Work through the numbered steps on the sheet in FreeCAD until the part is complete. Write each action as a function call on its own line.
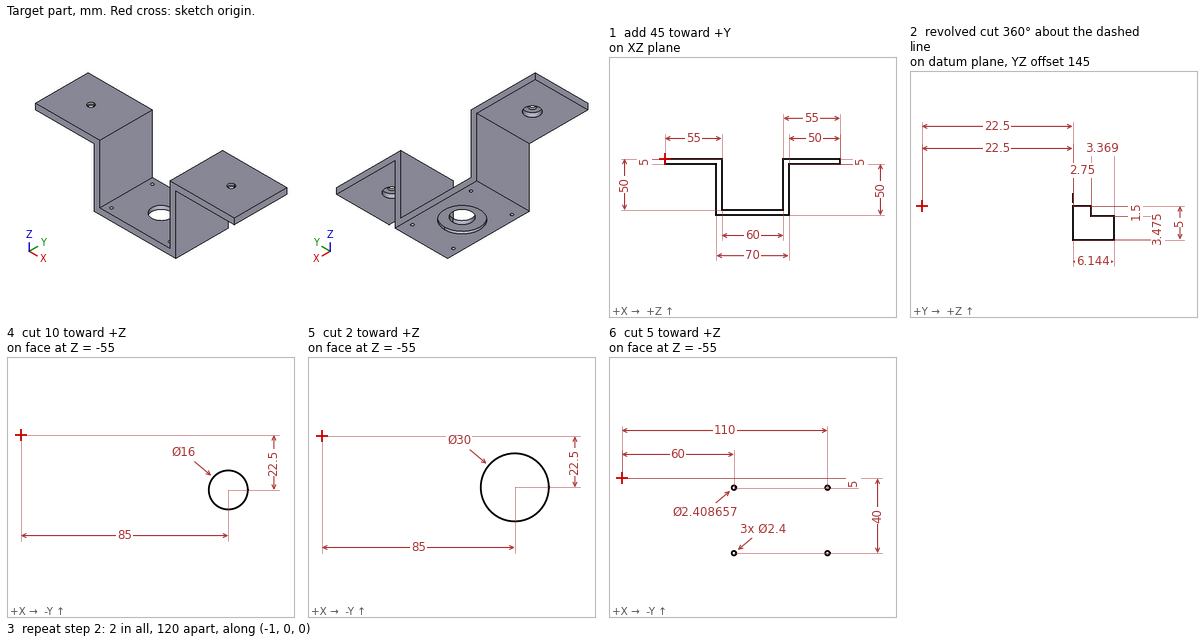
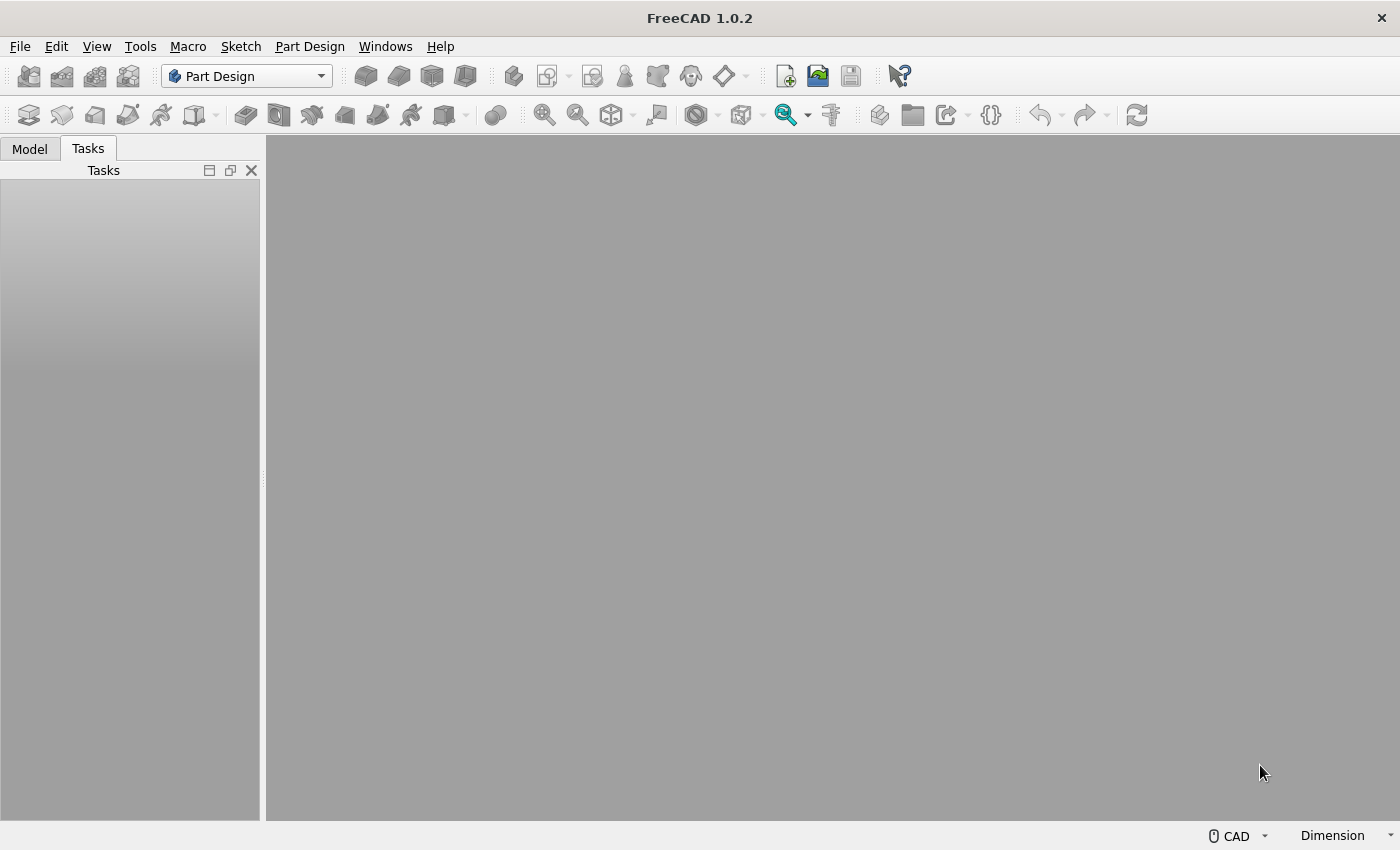
click(785, 76)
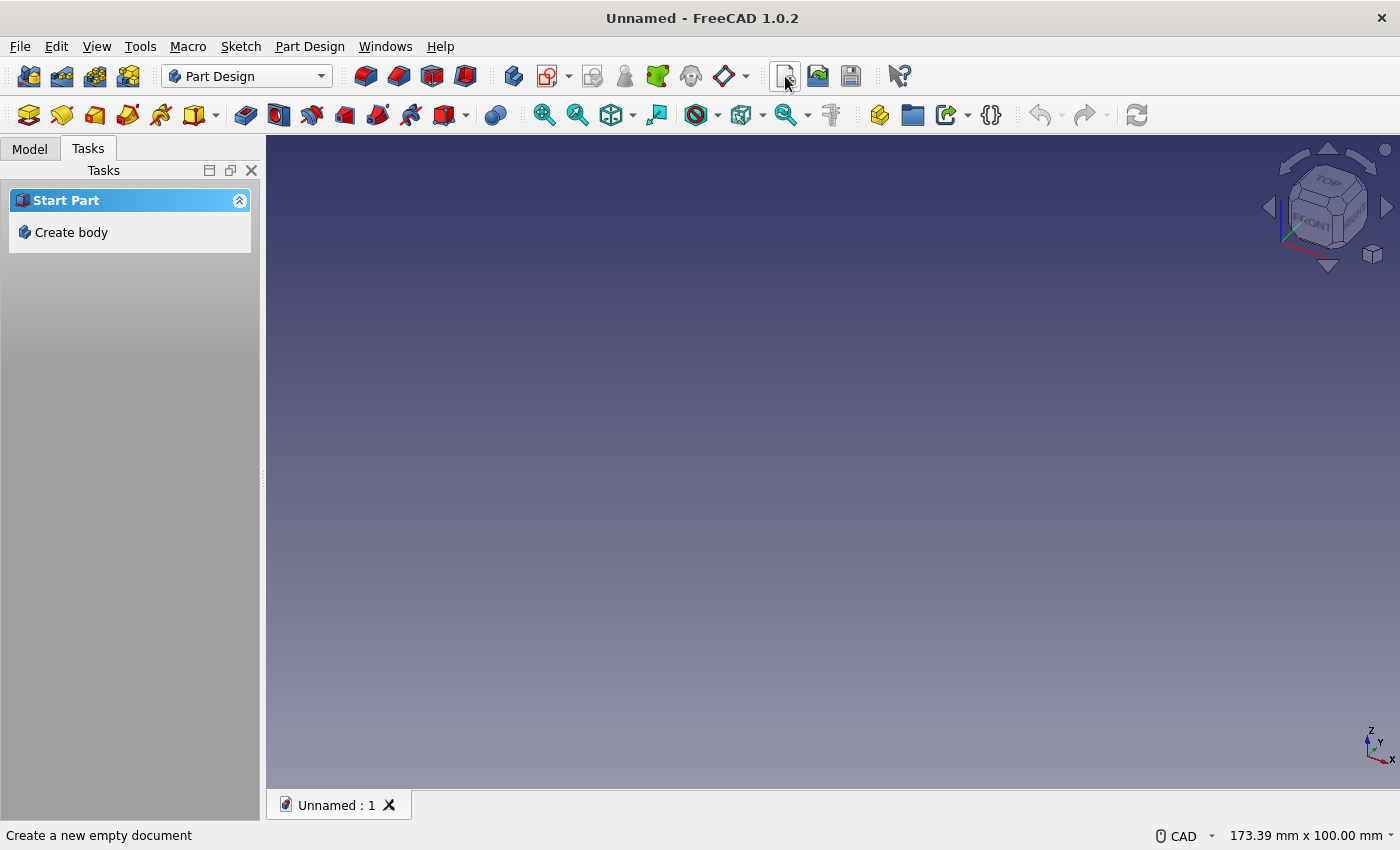
click(546, 76)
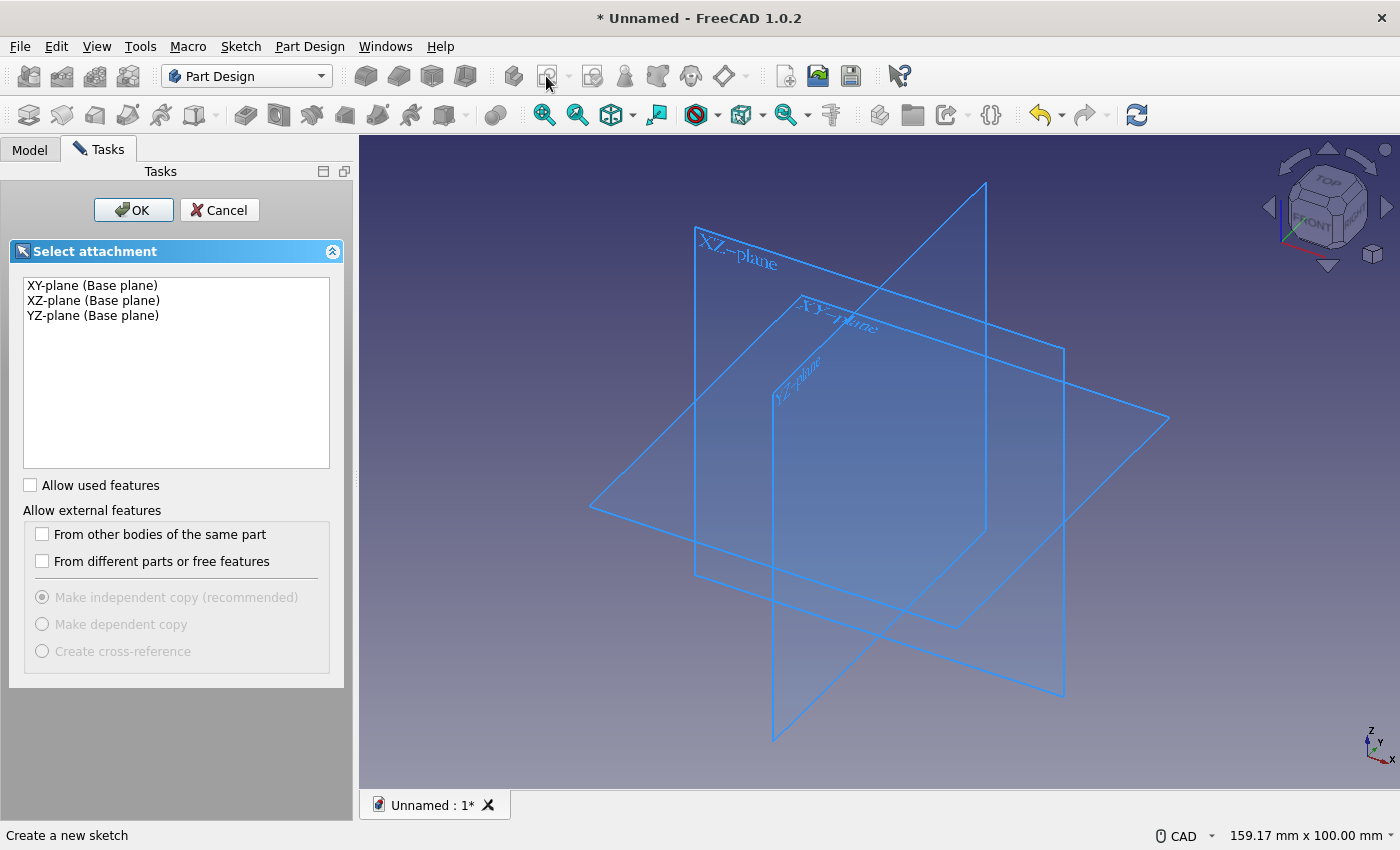
click(84, 300)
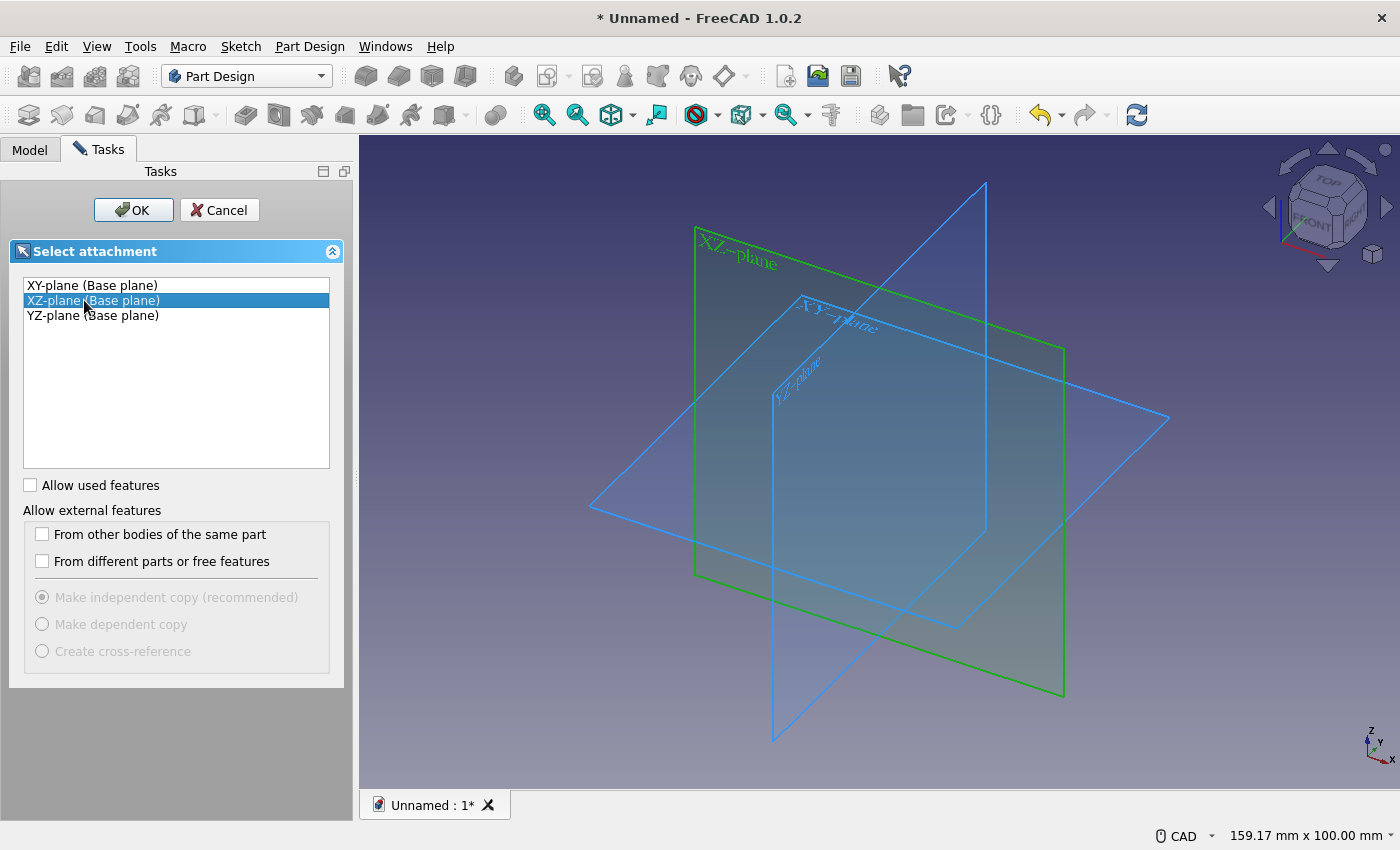
click(134, 210)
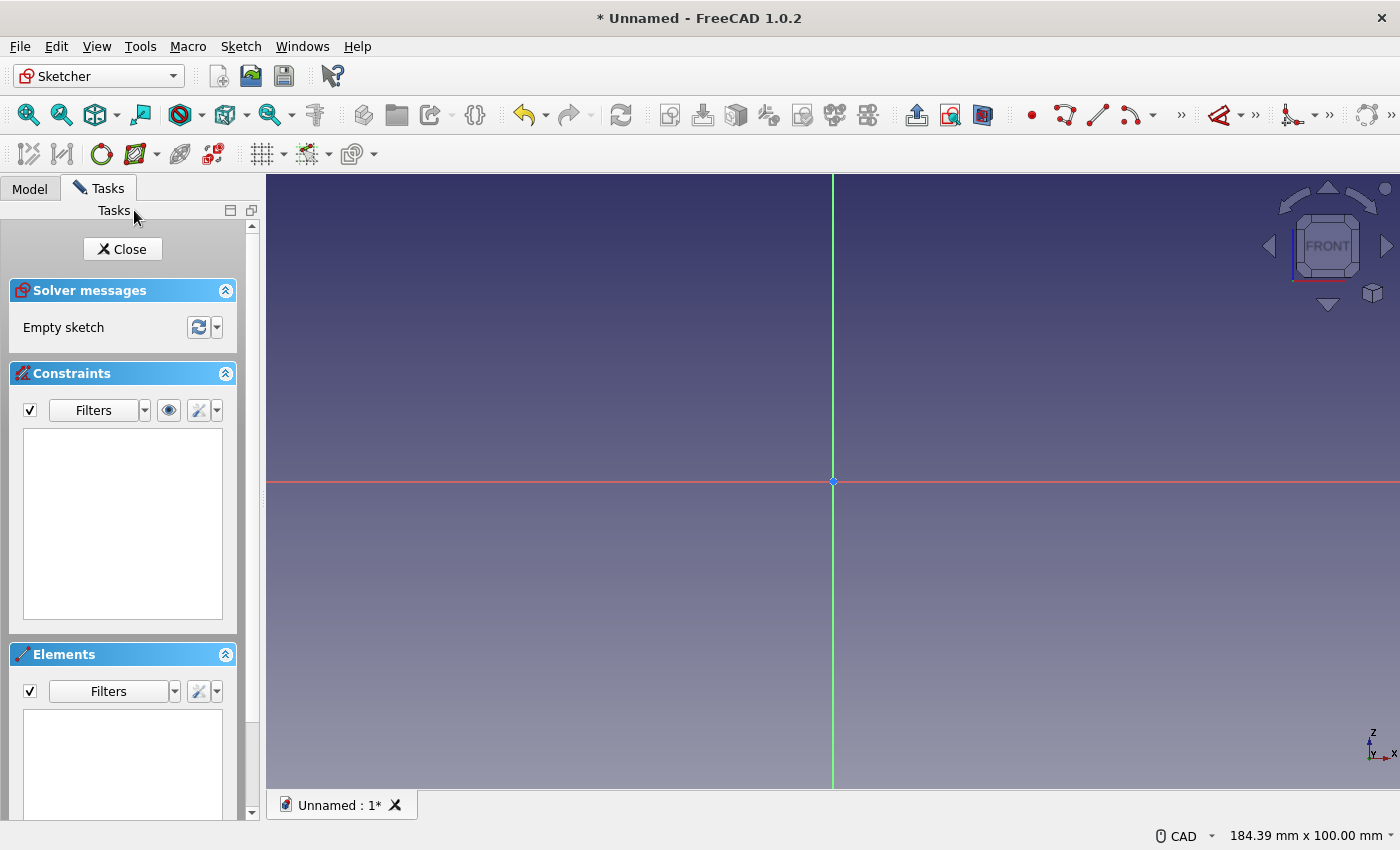
scroll(294, 276, down, 3)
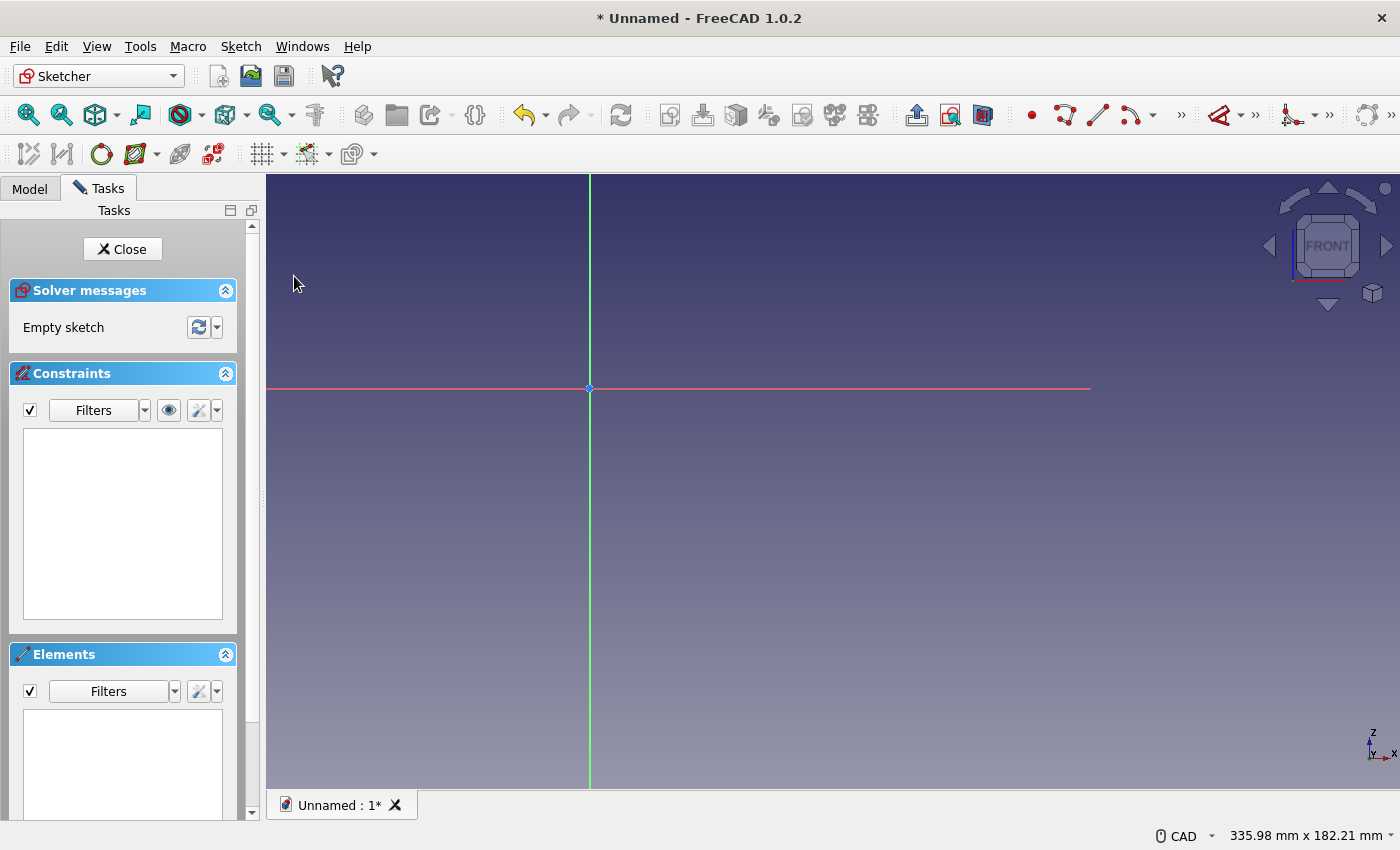
click(1065, 116)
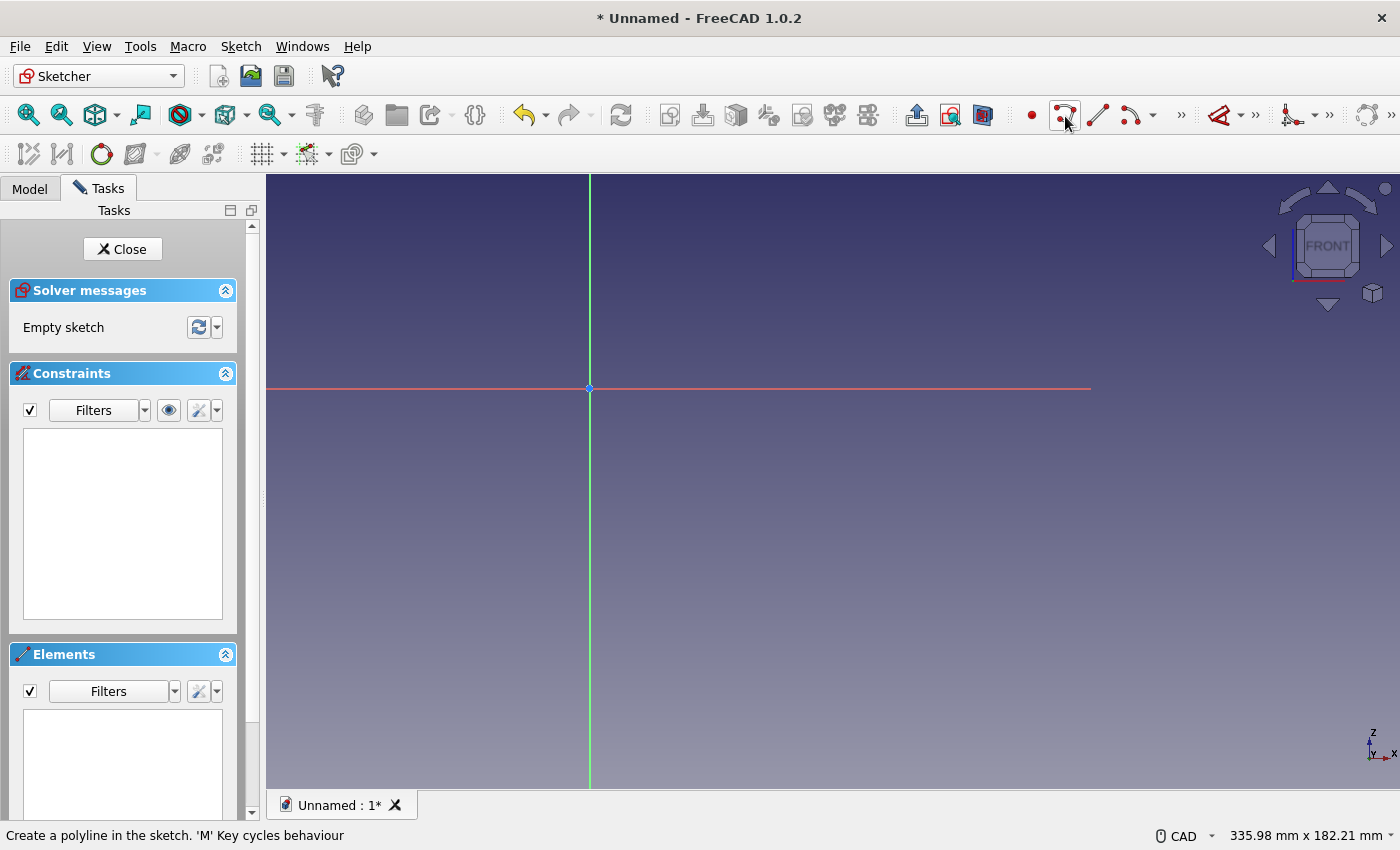
click(590, 389)
click(775, 398)
click(775, 558)
click(978, 558)
click(978, 389)
click(1164, 398)
click(1164, 406)
click(995, 406)
click(995, 574)
click(759, 574)
click(759, 406)
click(599, 406)
click(590, 389)
key(Escape)
key(Escape)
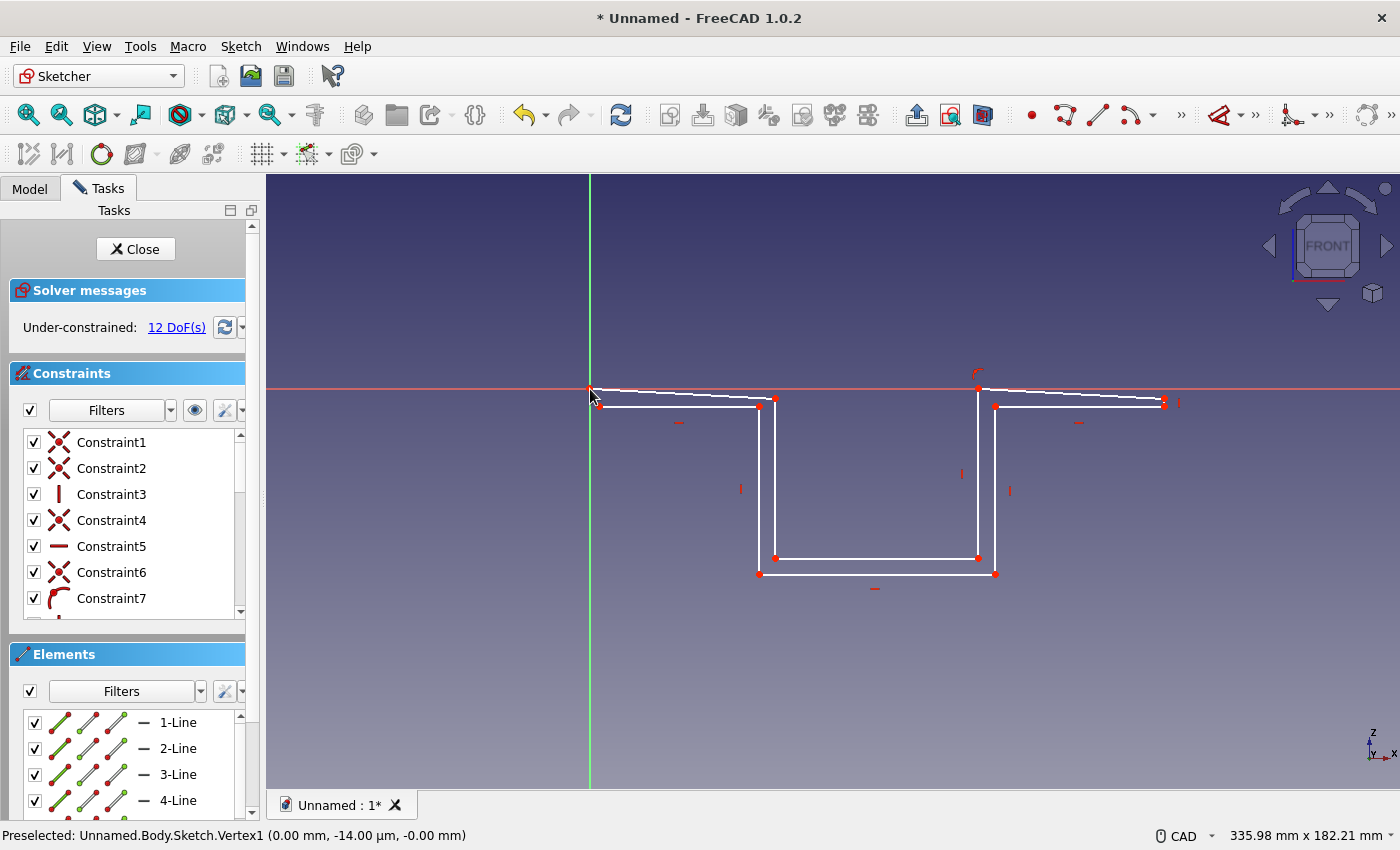
click(645, 392)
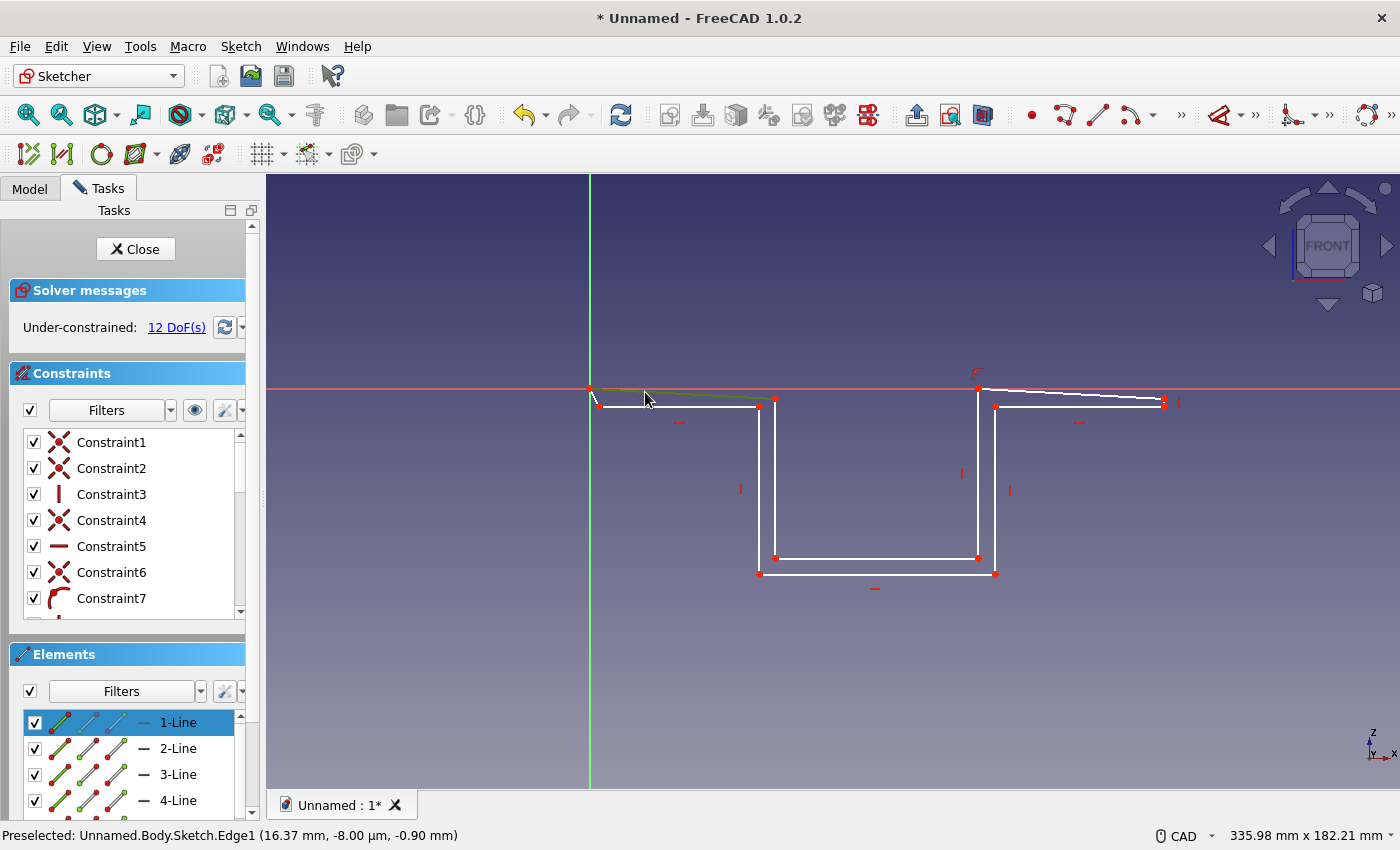
key(h)